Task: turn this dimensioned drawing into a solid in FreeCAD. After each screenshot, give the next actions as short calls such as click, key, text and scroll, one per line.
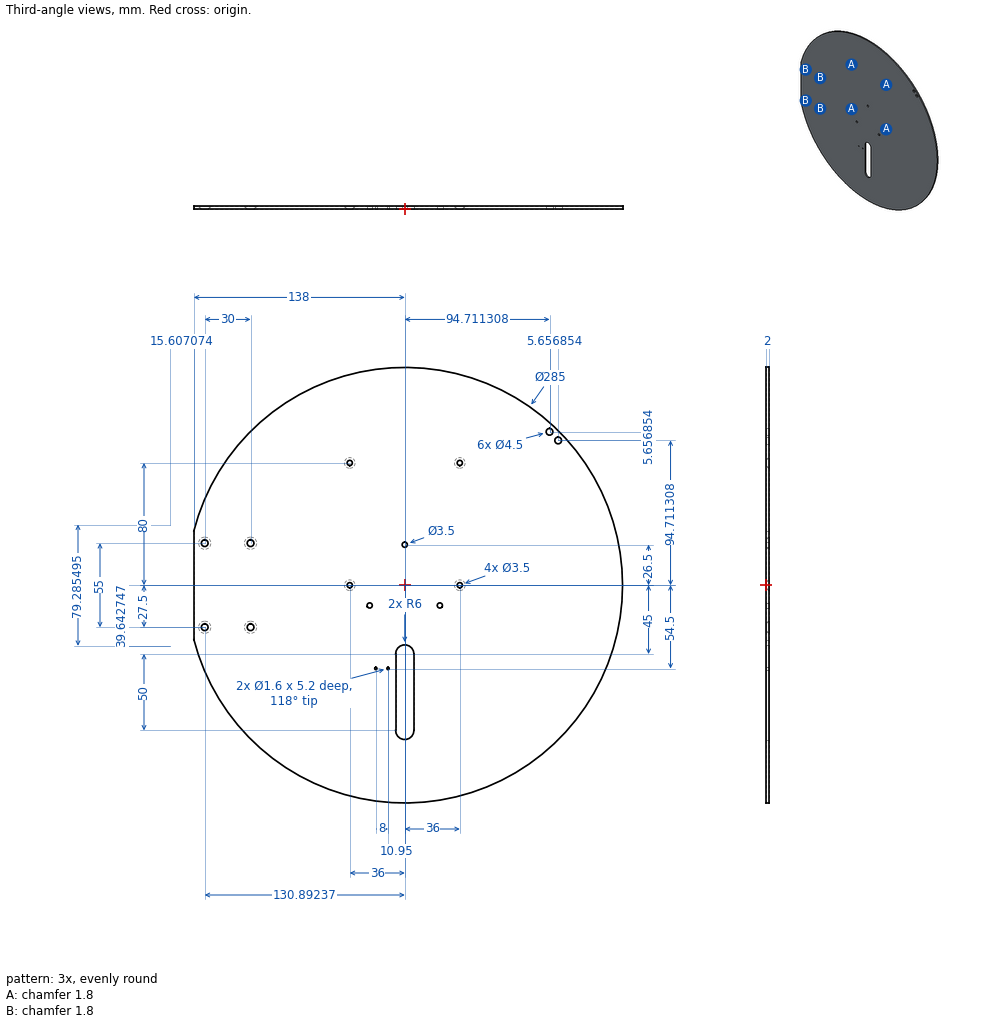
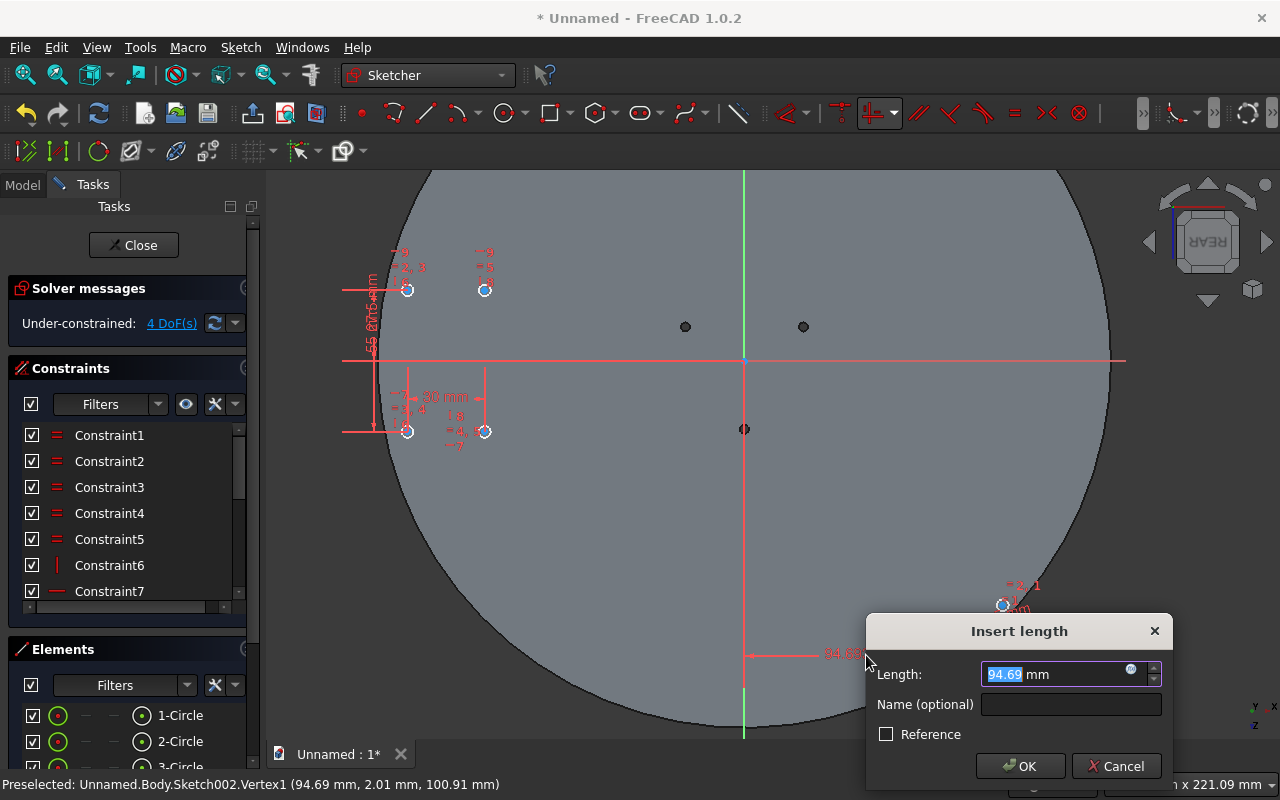
text(94.711308)
key(Return)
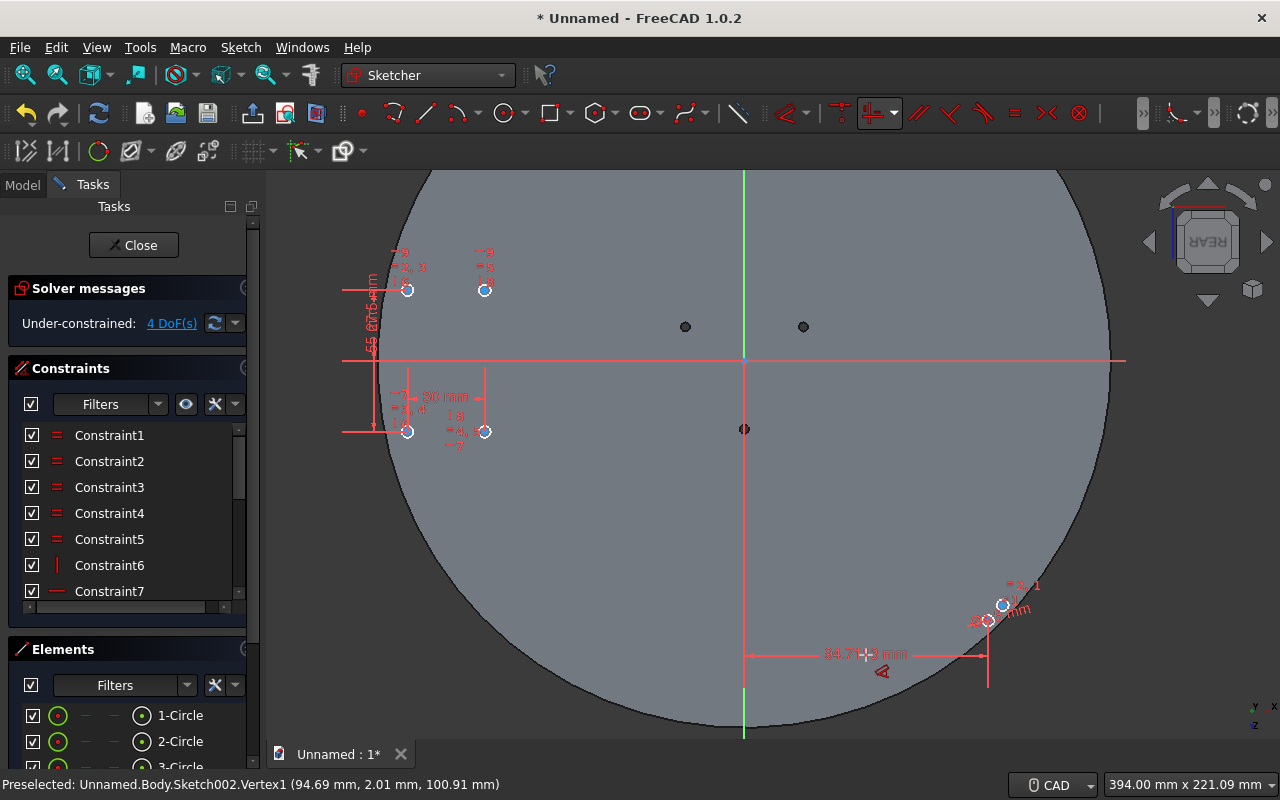
click(1003, 605)
click(1037, 483)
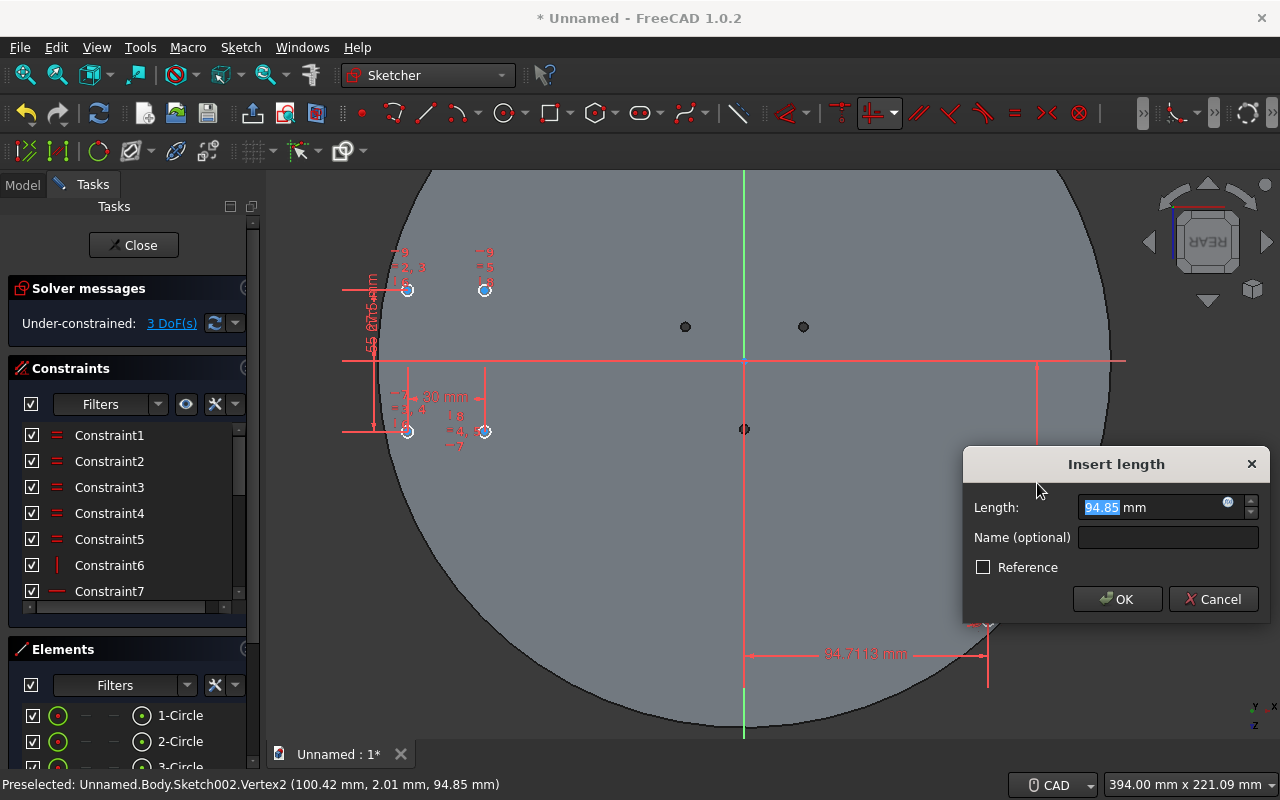
text(94.711308)
key(Return)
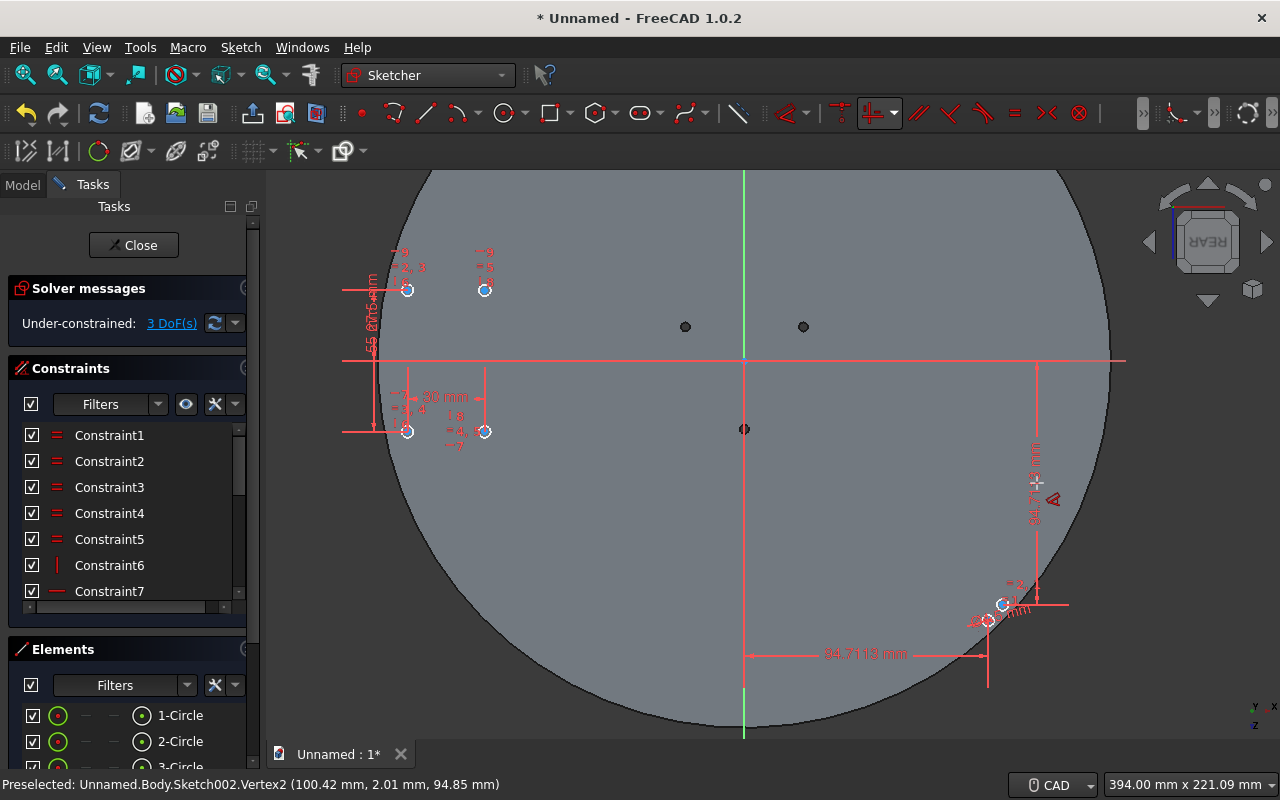
click(408, 290)
click(576, 256)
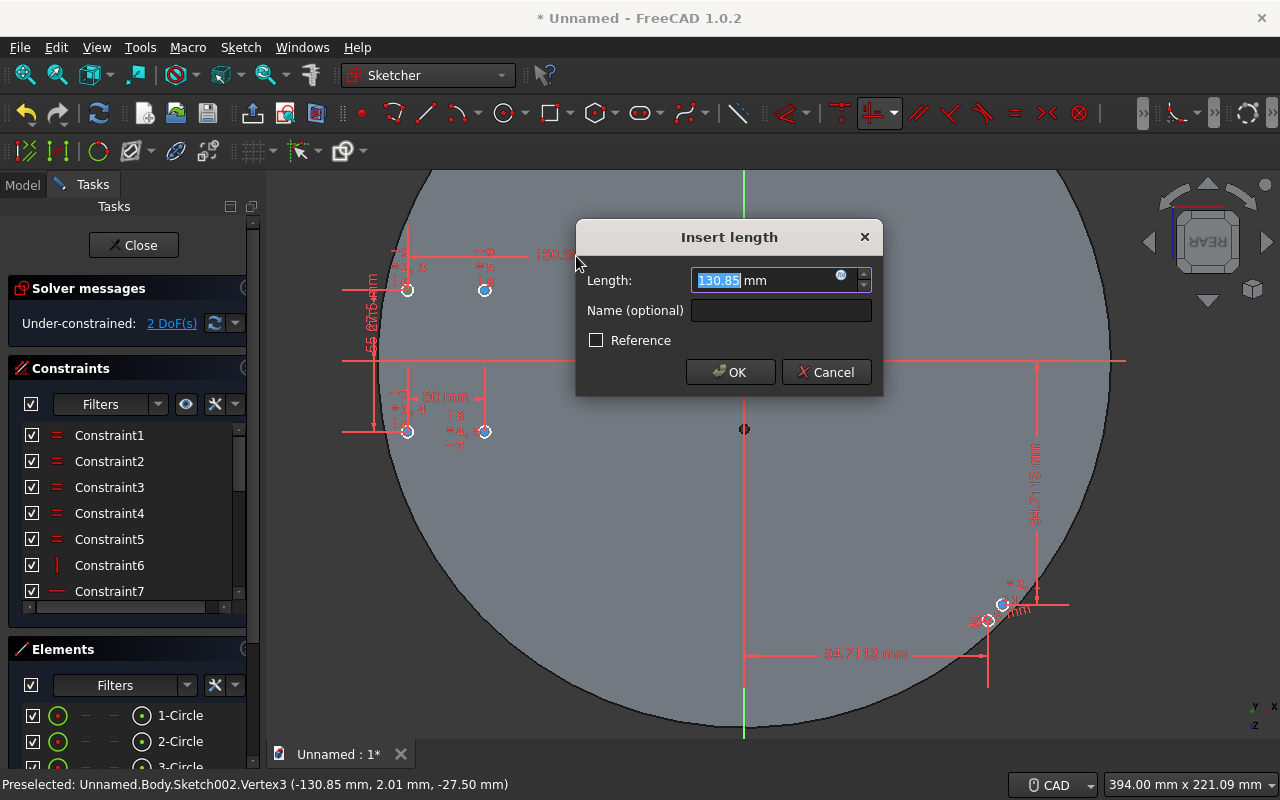
text(130.89237)
key(Return)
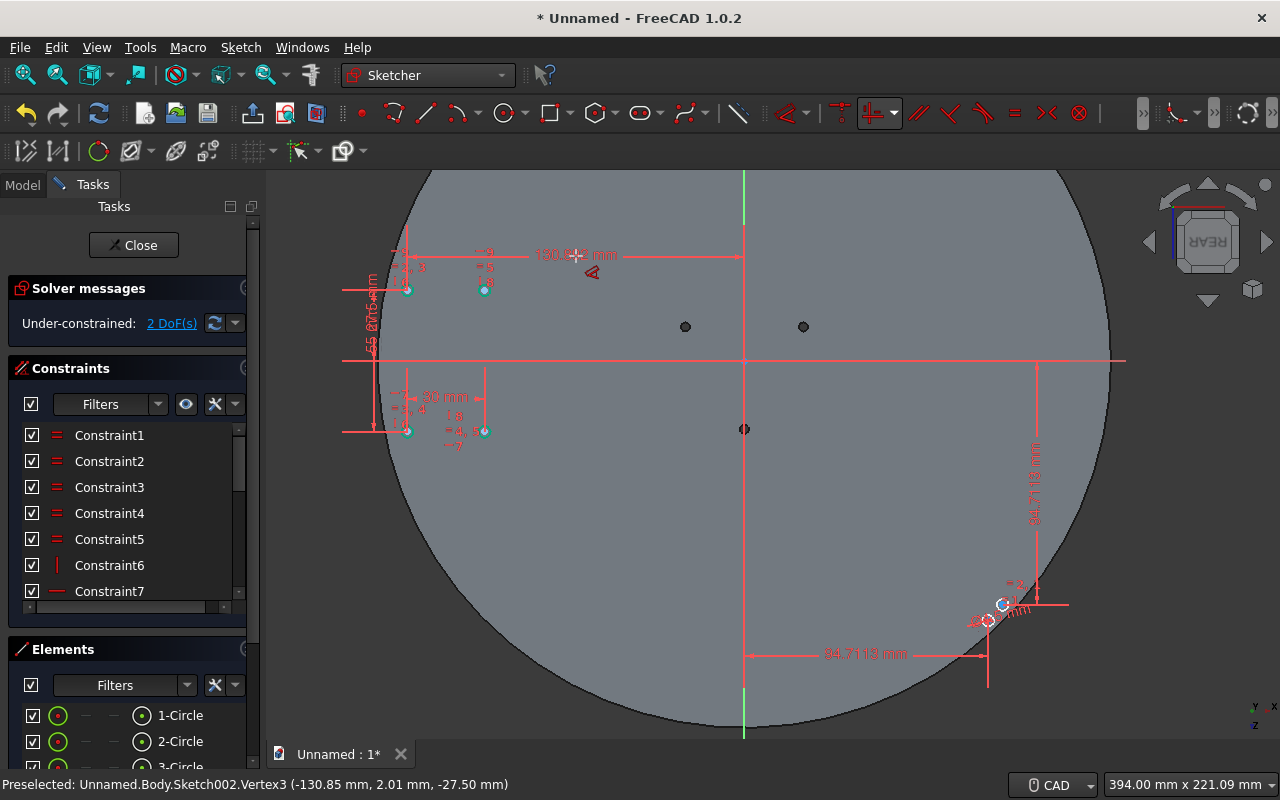
scroll(988, 621, up, 6)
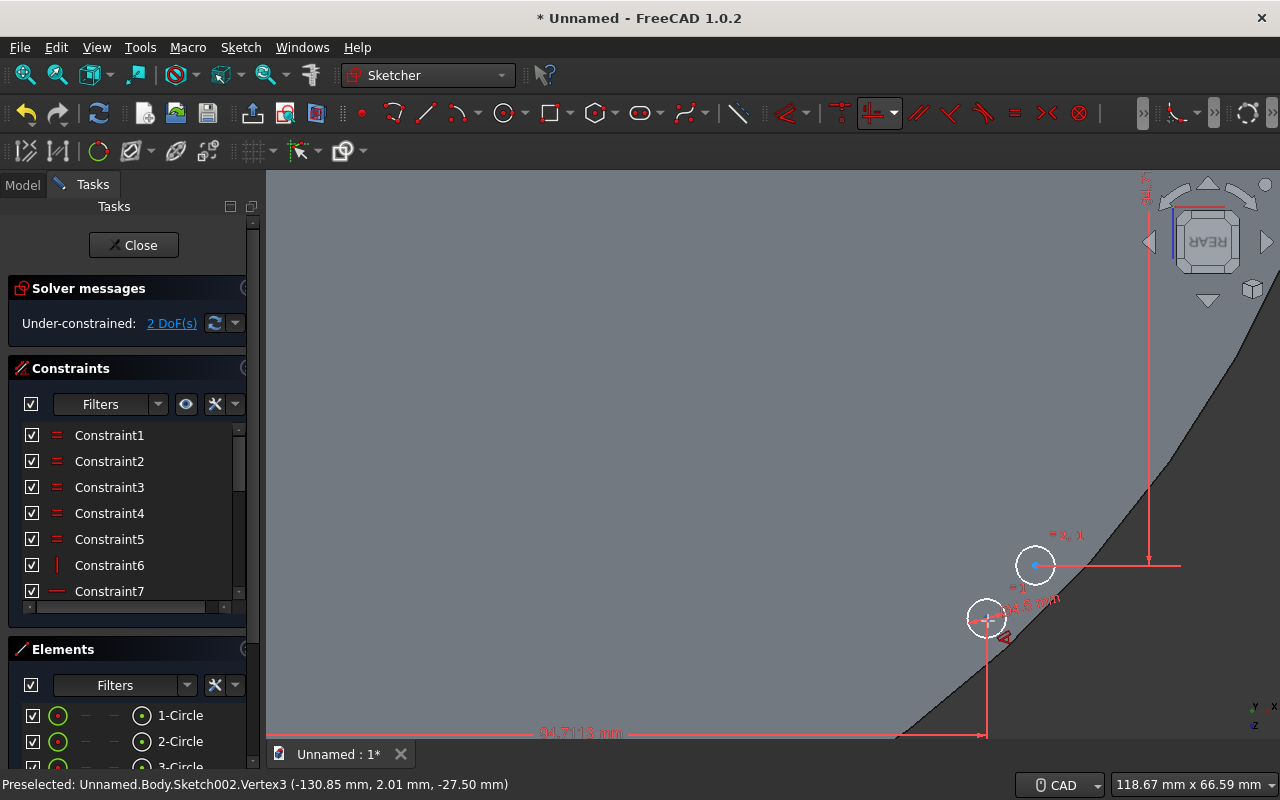
click(987, 618)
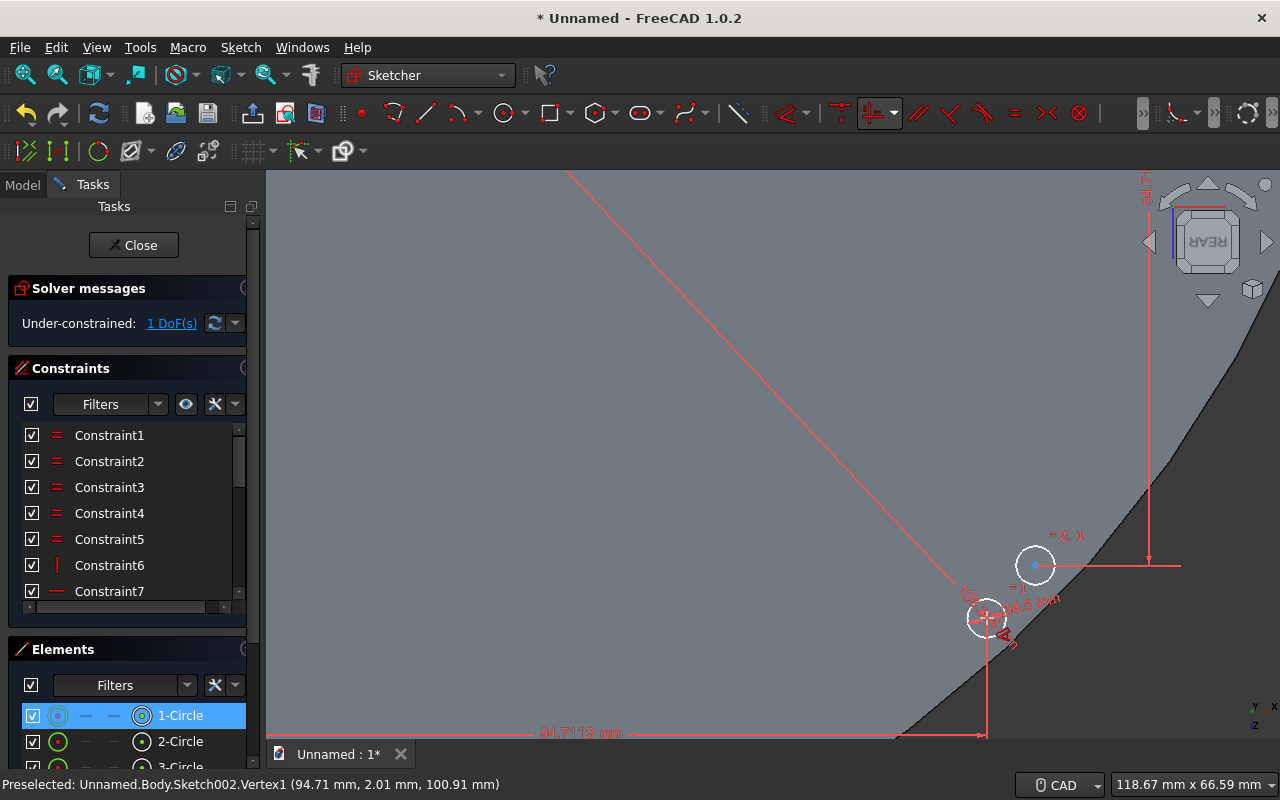
click(1035, 566)
click(1011, 652)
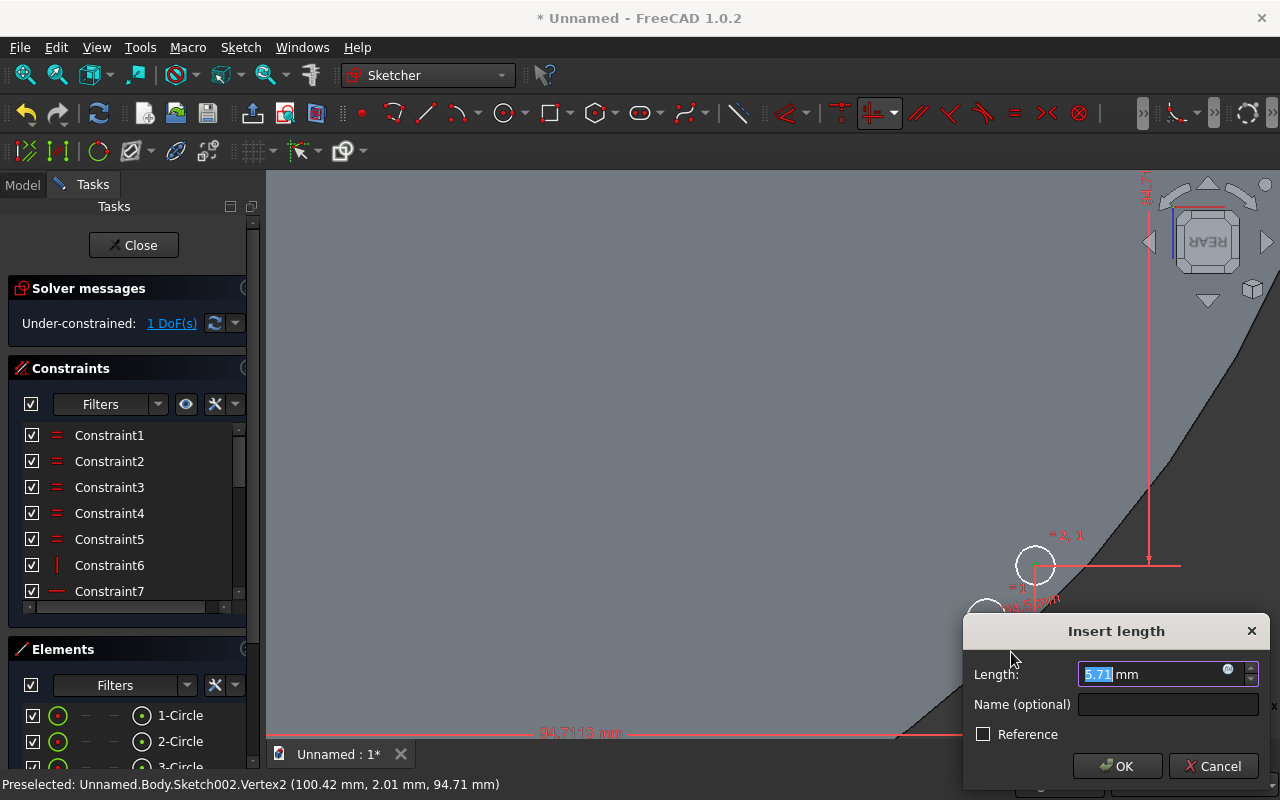
text(5.656854)
key(Return)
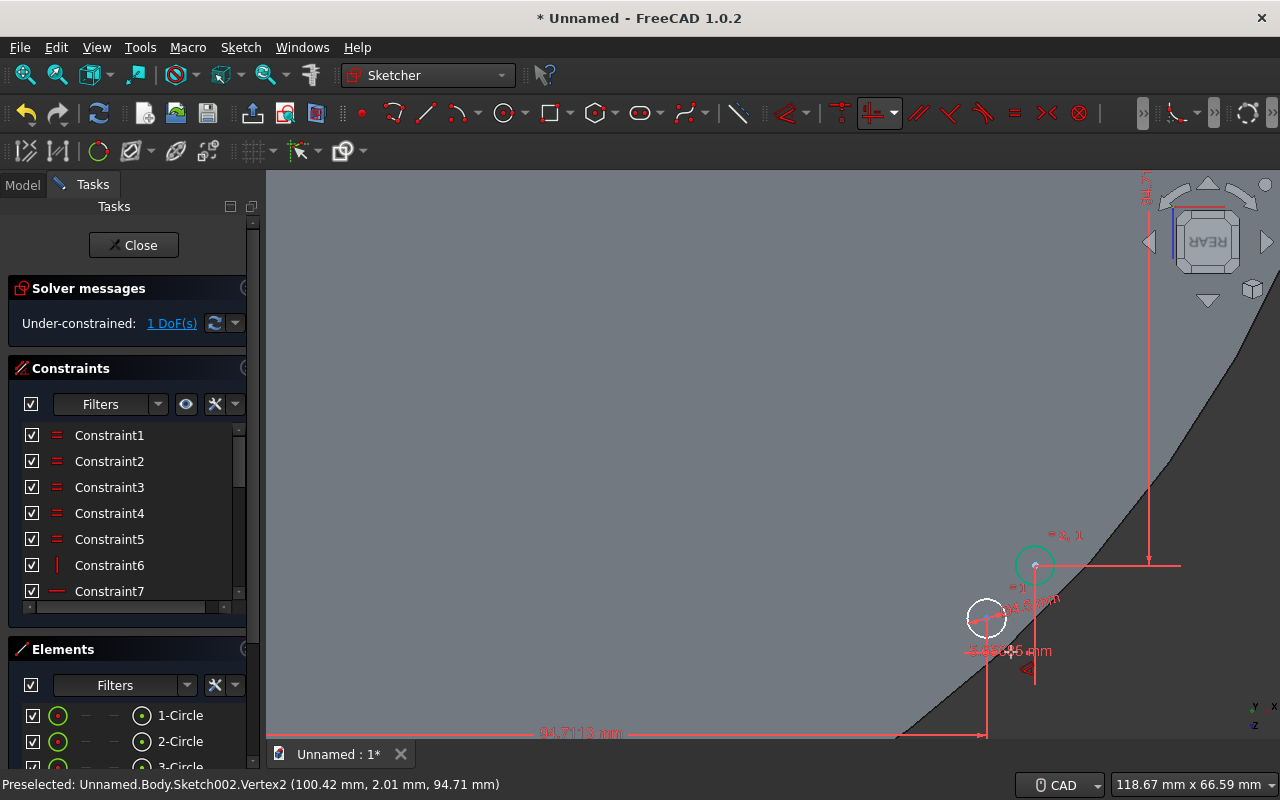
click(987, 618)